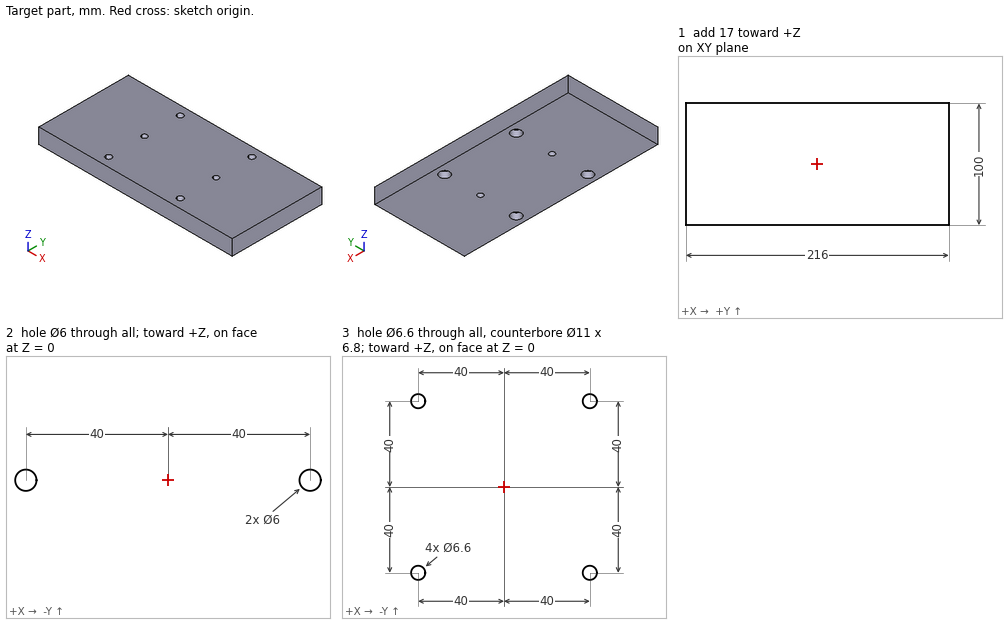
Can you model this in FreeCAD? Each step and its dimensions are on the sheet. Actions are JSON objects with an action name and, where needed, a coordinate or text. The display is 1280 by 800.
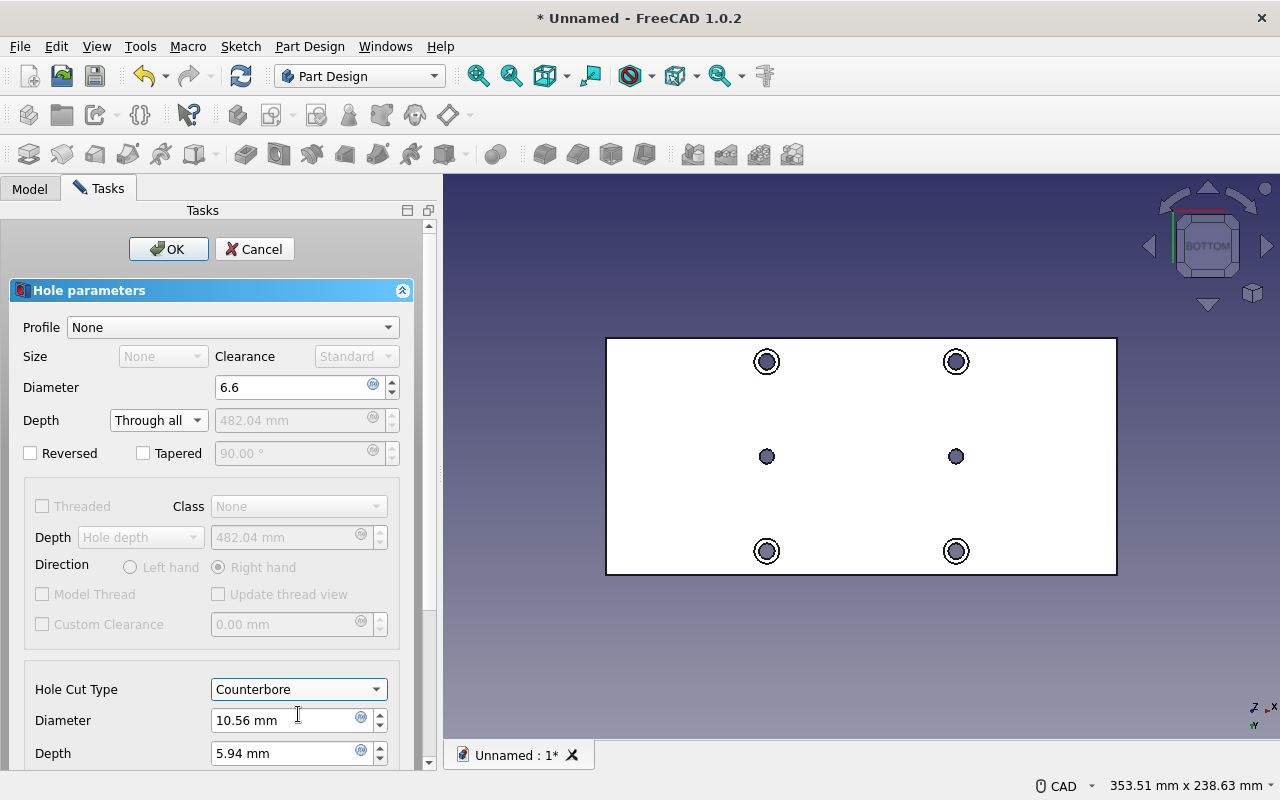
{"action": "triple_click", "coordinate": [292, 720]}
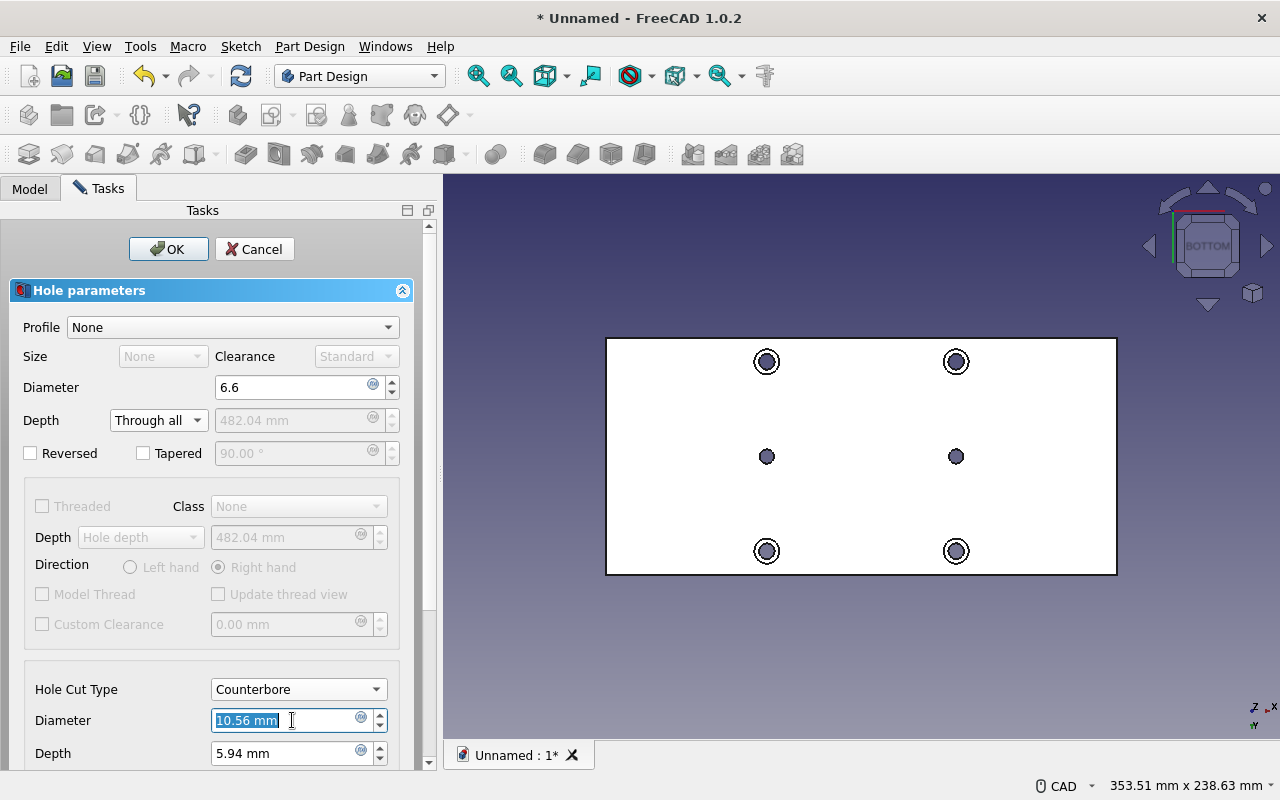
{"action": "type", "text": "11"}
{"action": "key", "text": "Tab"}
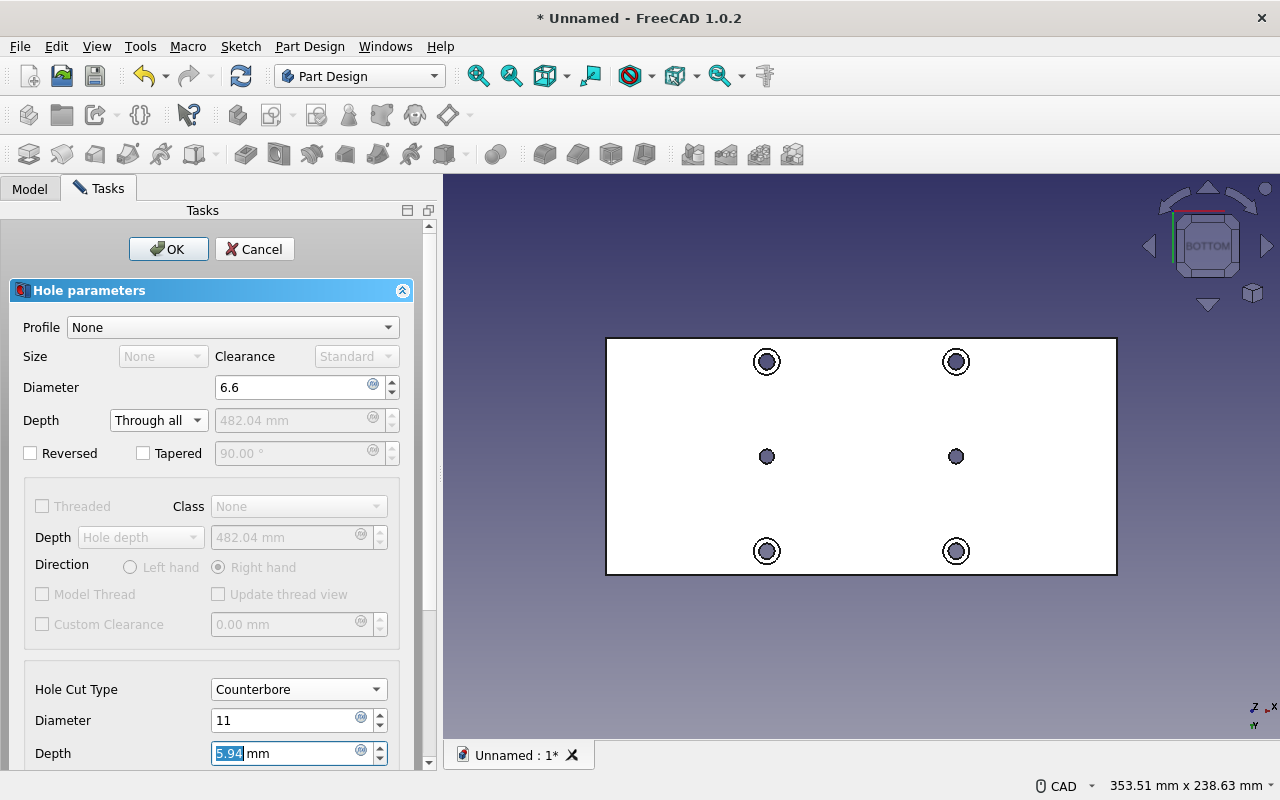
{"action": "type", "text": "6.8"}
{"action": "key", "text": "Tab"}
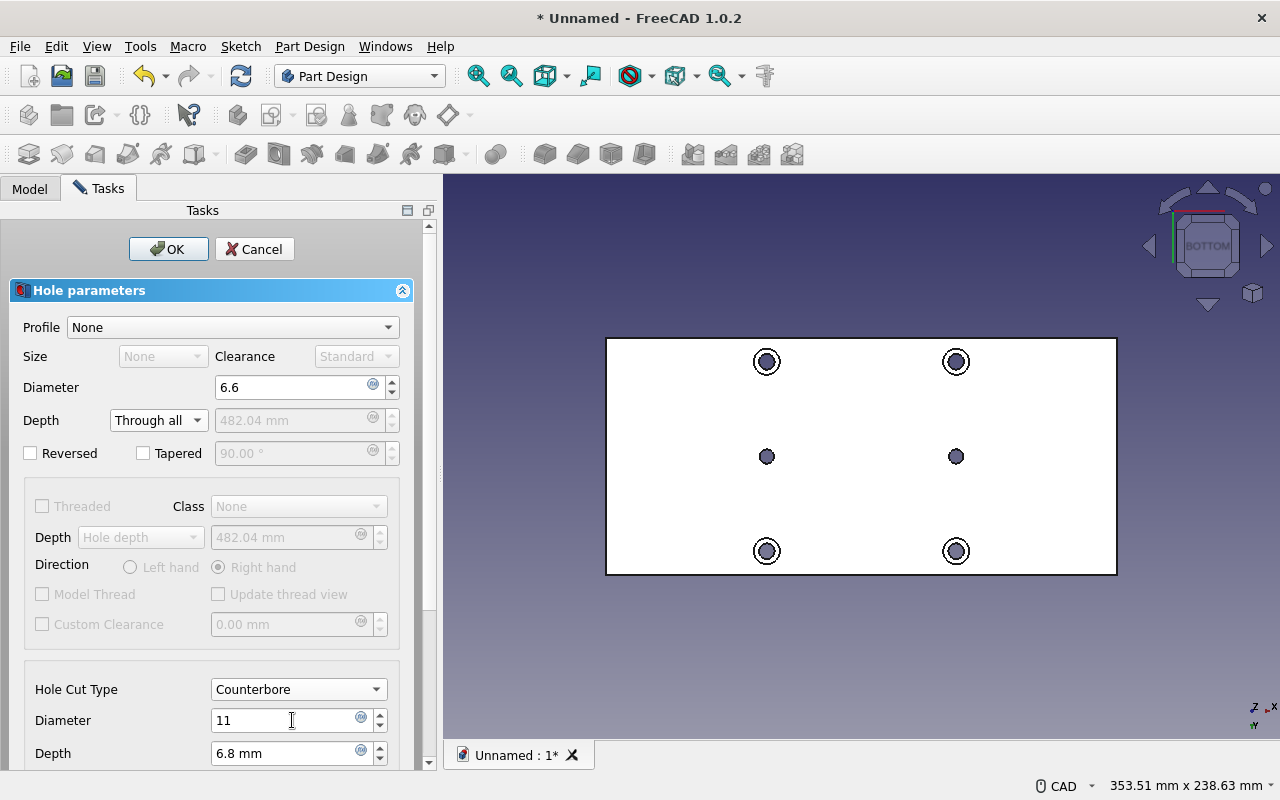
{"action": "left_click", "coordinate": [169, 249]}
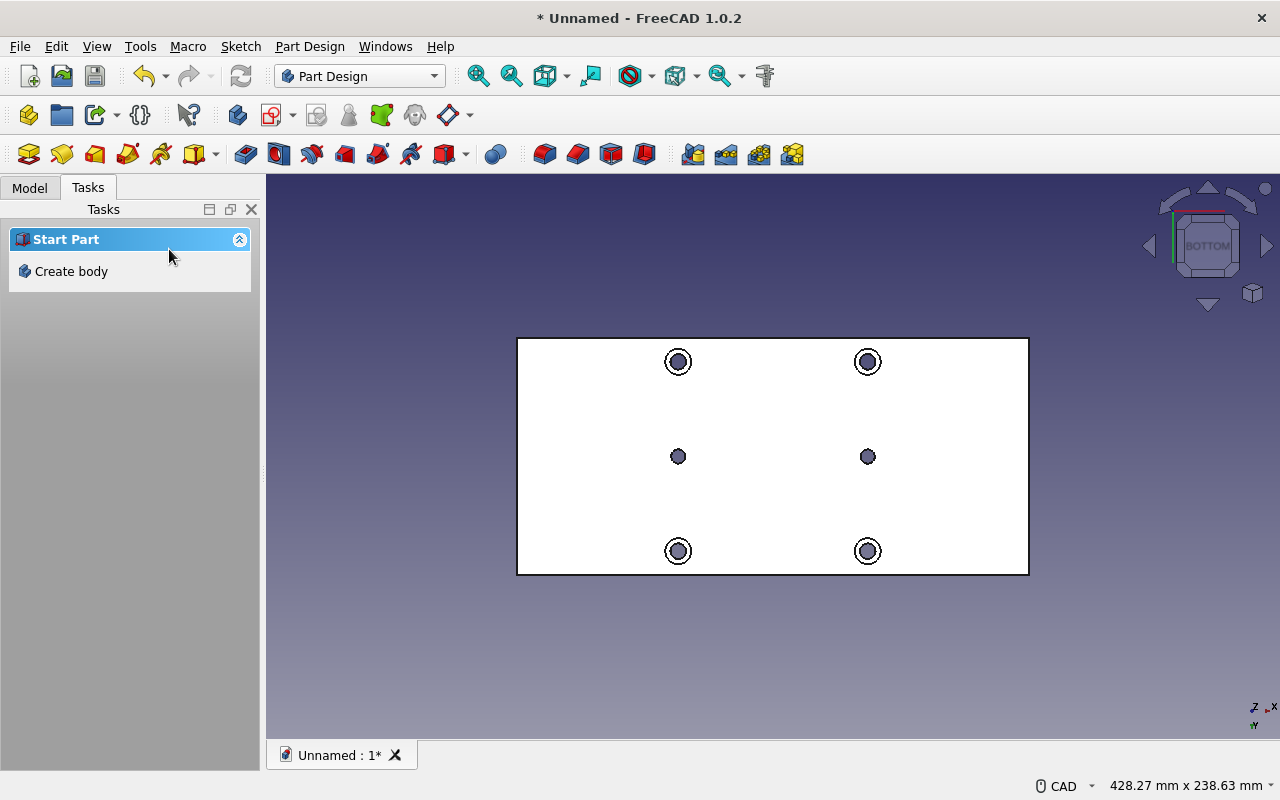
{"action": "key", "text": "0"}